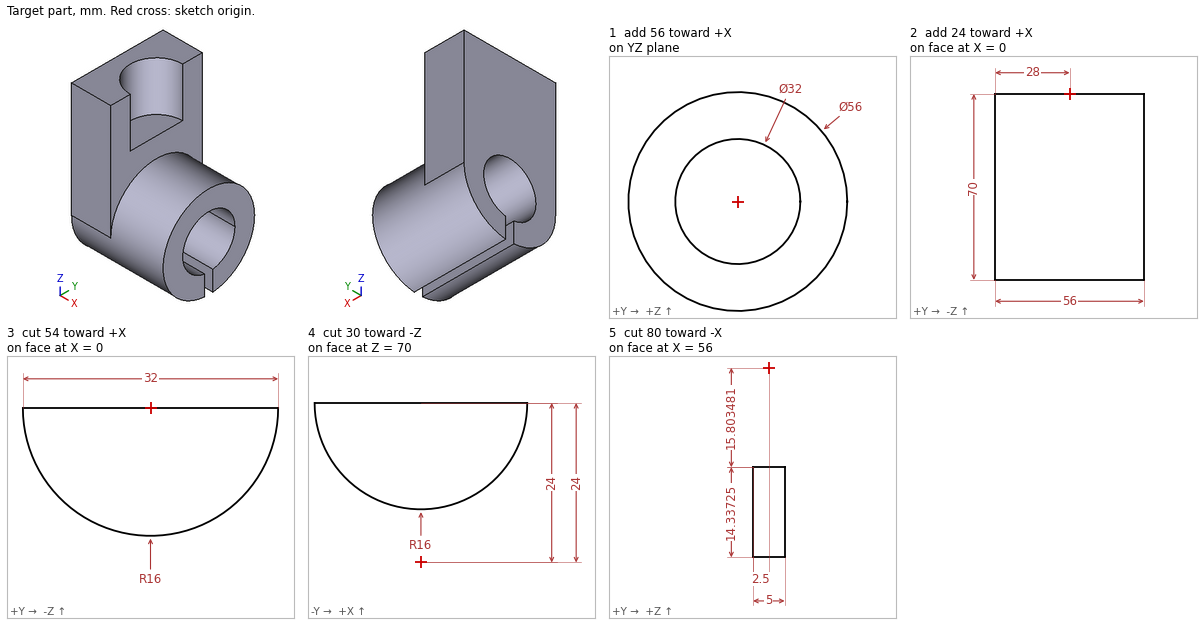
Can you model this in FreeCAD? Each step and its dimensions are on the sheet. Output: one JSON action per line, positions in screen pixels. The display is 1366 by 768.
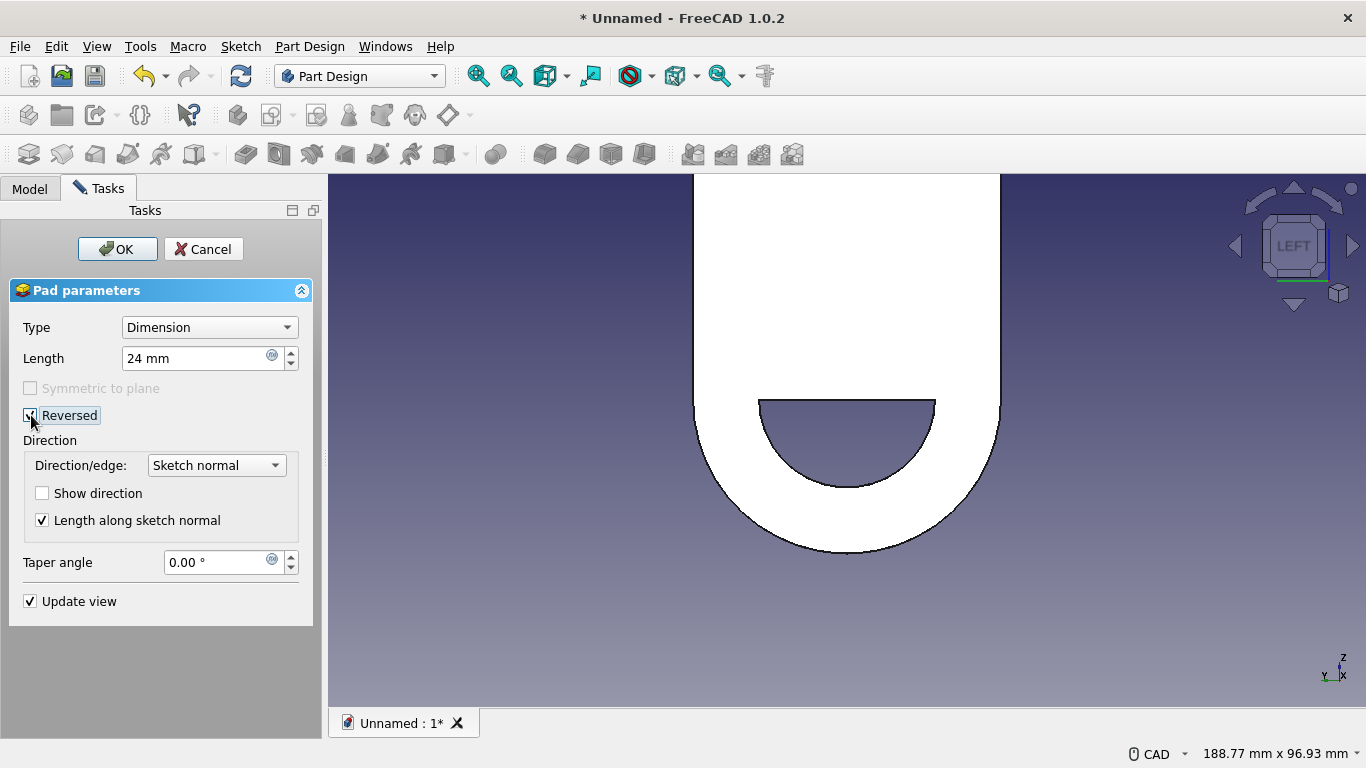
{"action": "left_click", "coordinate": [118, 249]}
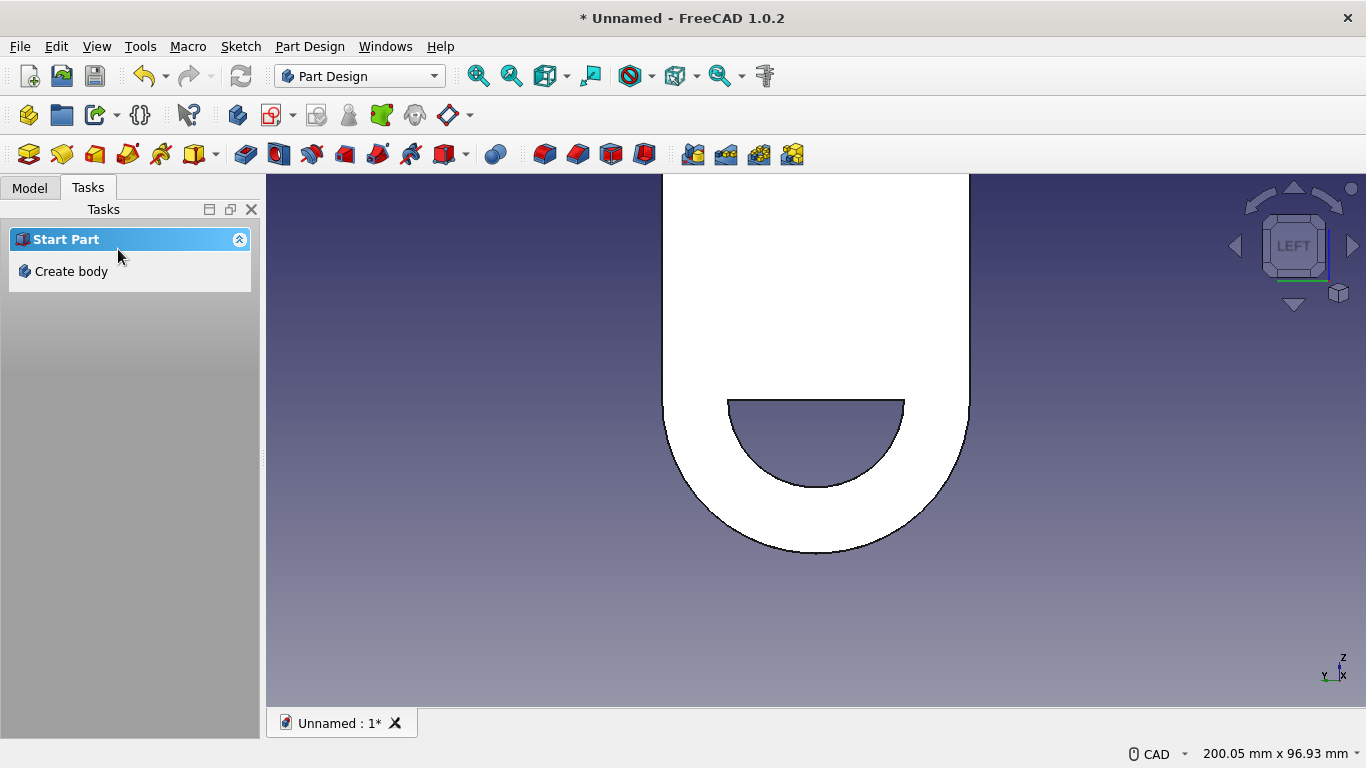
{"action": "left_click", "coordinate": [479, 76]}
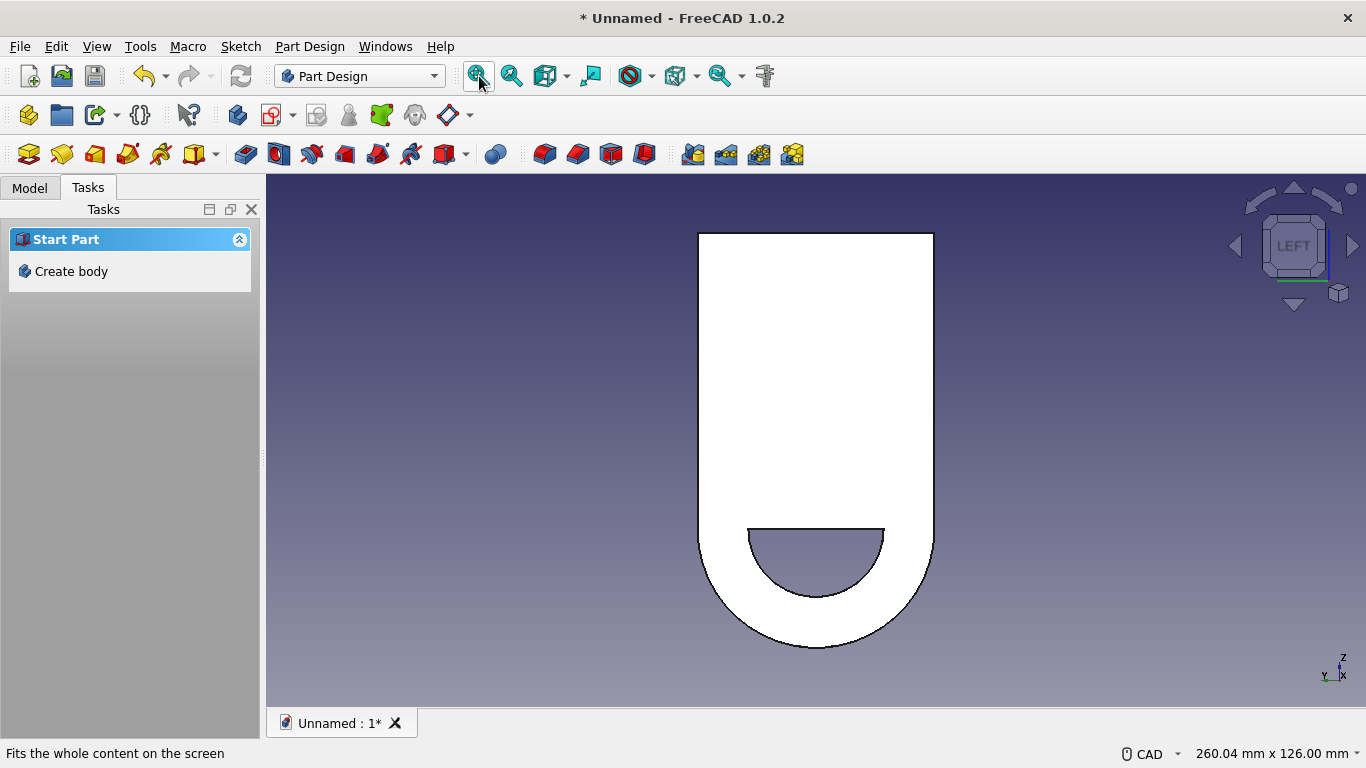
{"action": "left_click", "coordinate": [816, 380]}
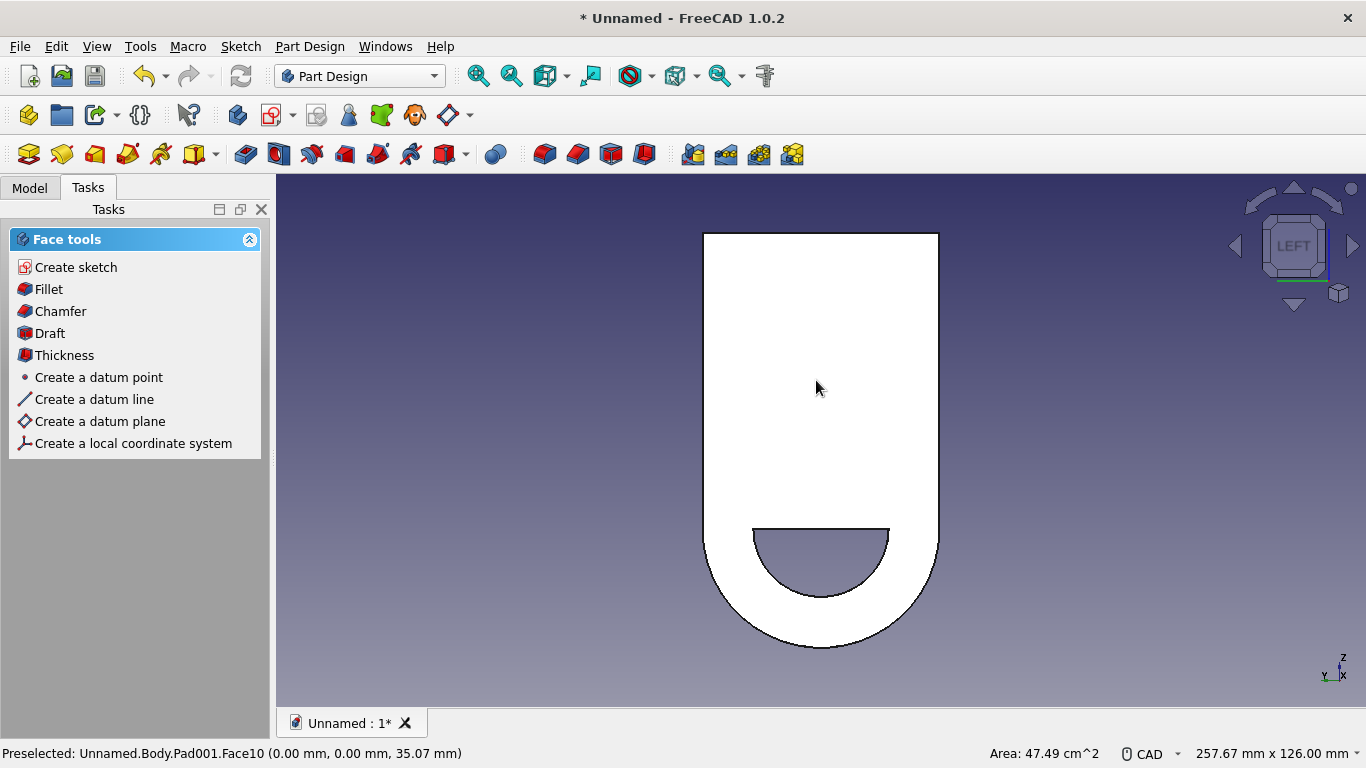
{"action": "left_click", "coordinate": [270, 116]}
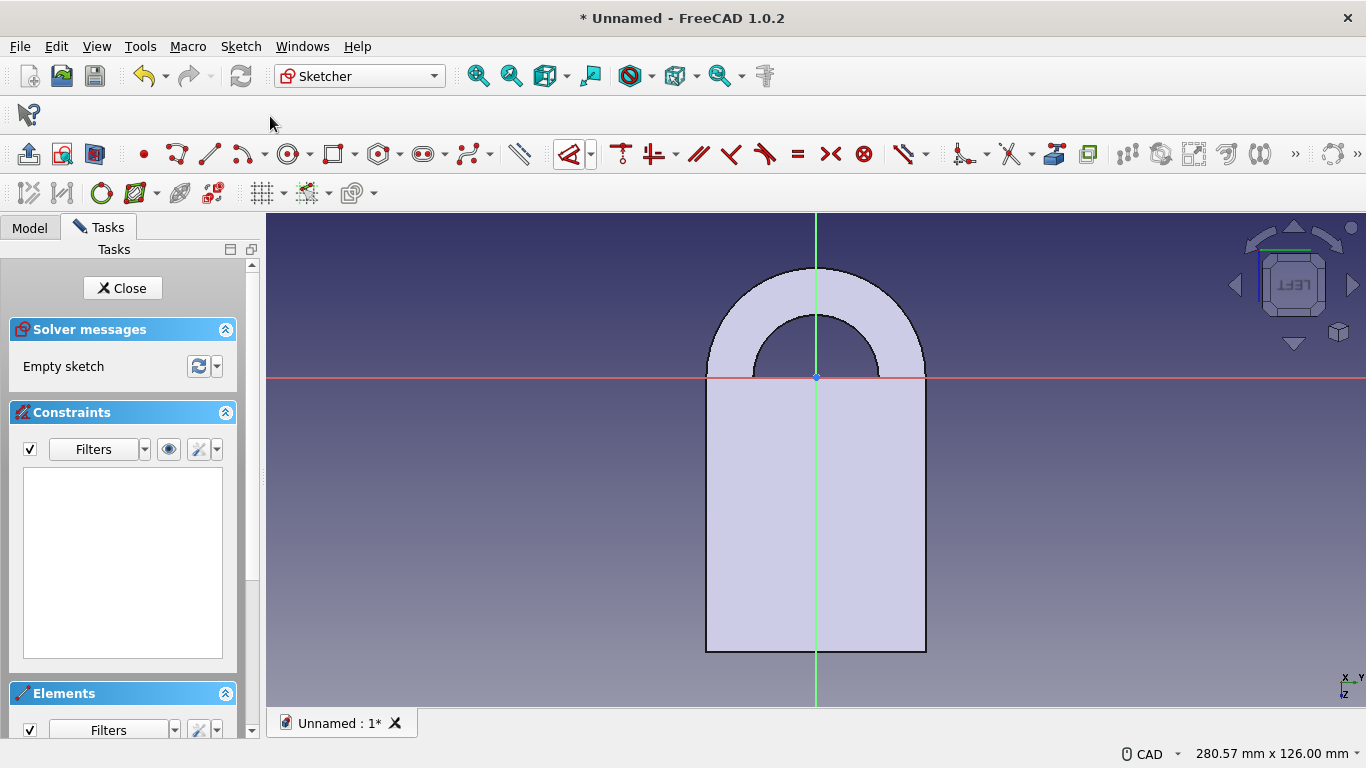
{"action": "scroll", "coordinate": [833, 396], "scroll_direction": "up", "scroll_amount": 8}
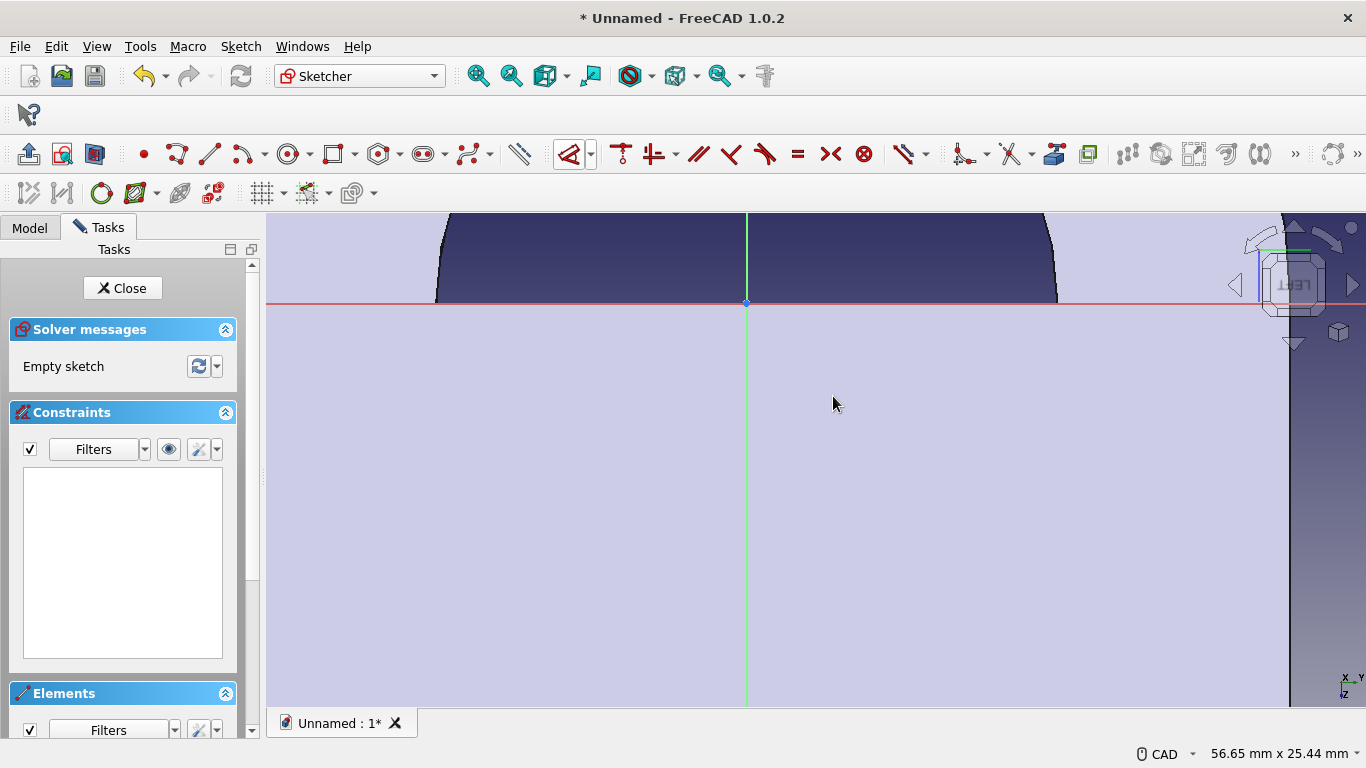
{"action": "left_click", "coordinate": [210, 154]}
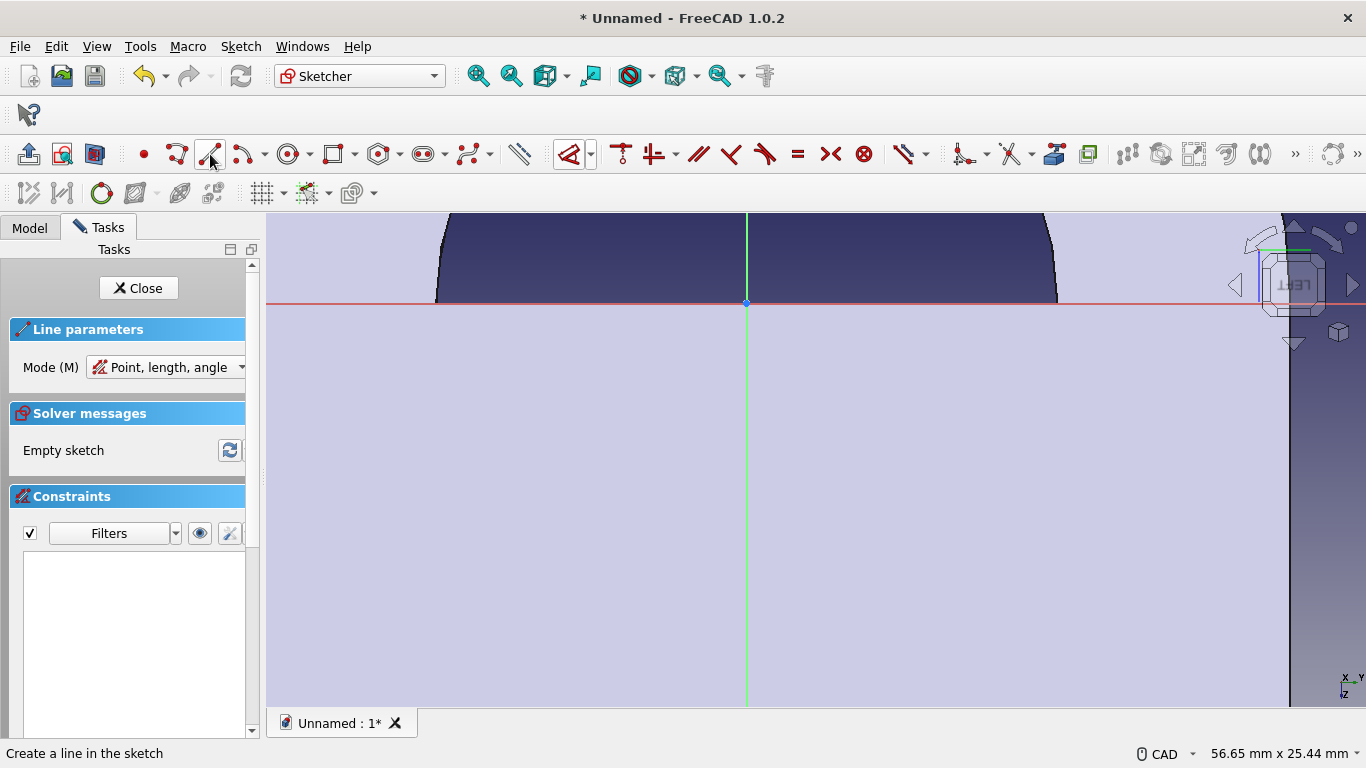
{"action": "left_click", "coordinate": [1057, 304]}
{"action": "left_click", "coordinate": [436, 313]}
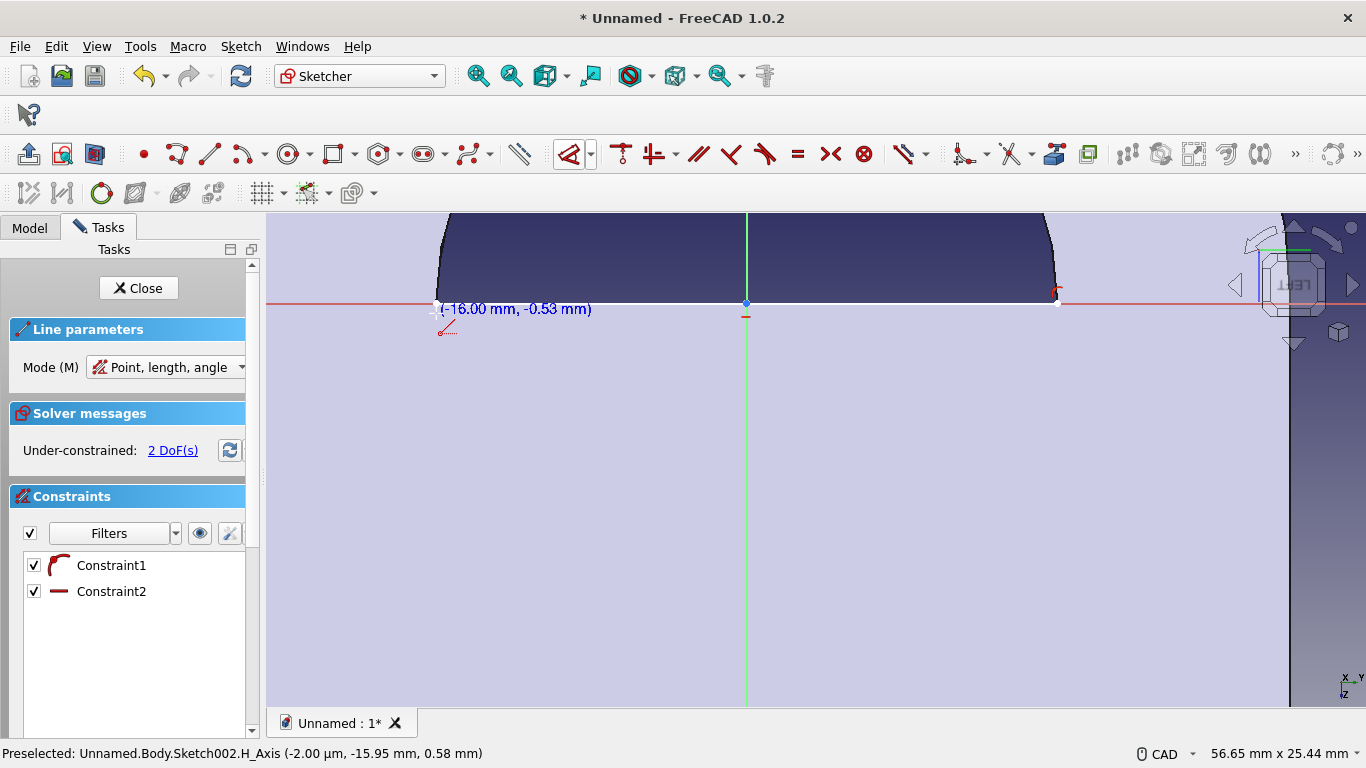
{"action": "left_click", "coordinate": [264, 154]}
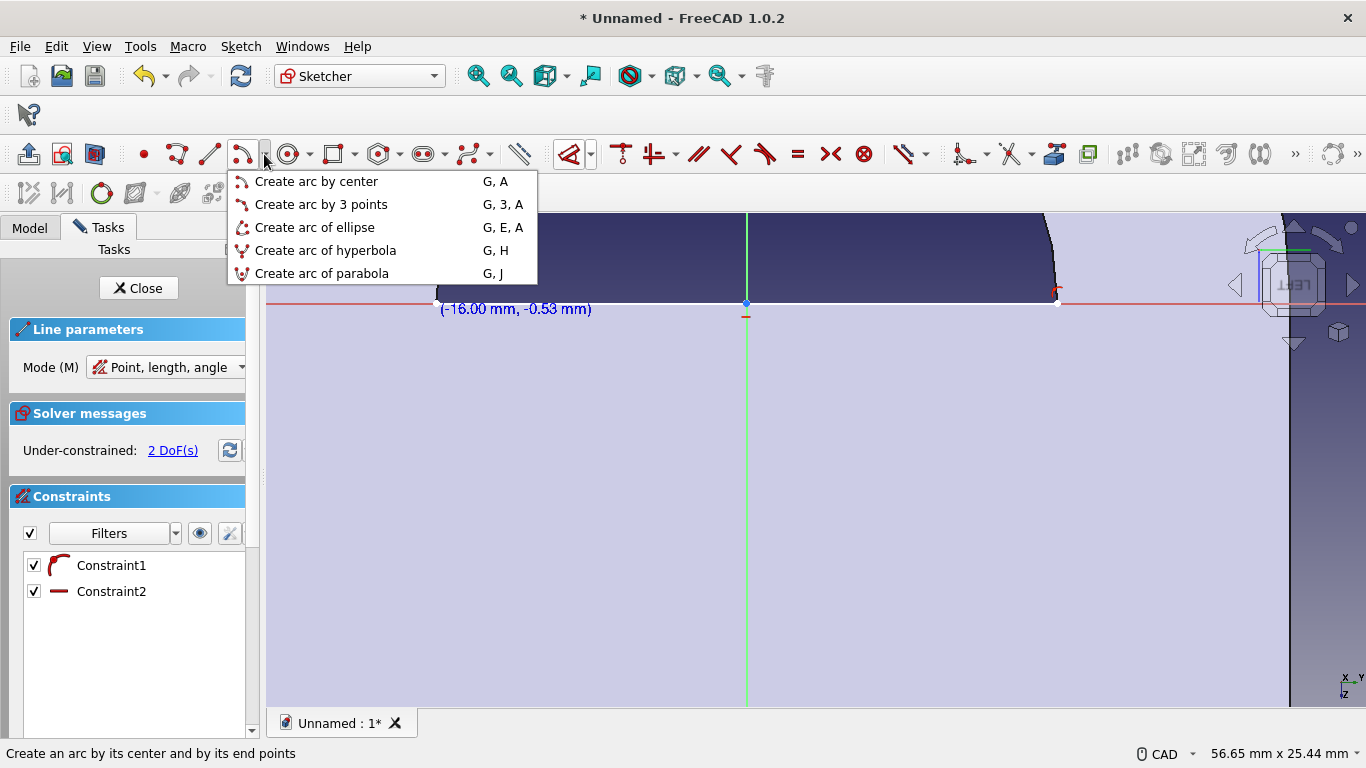
{"action": "left_click", "coordinate": [382, 204]}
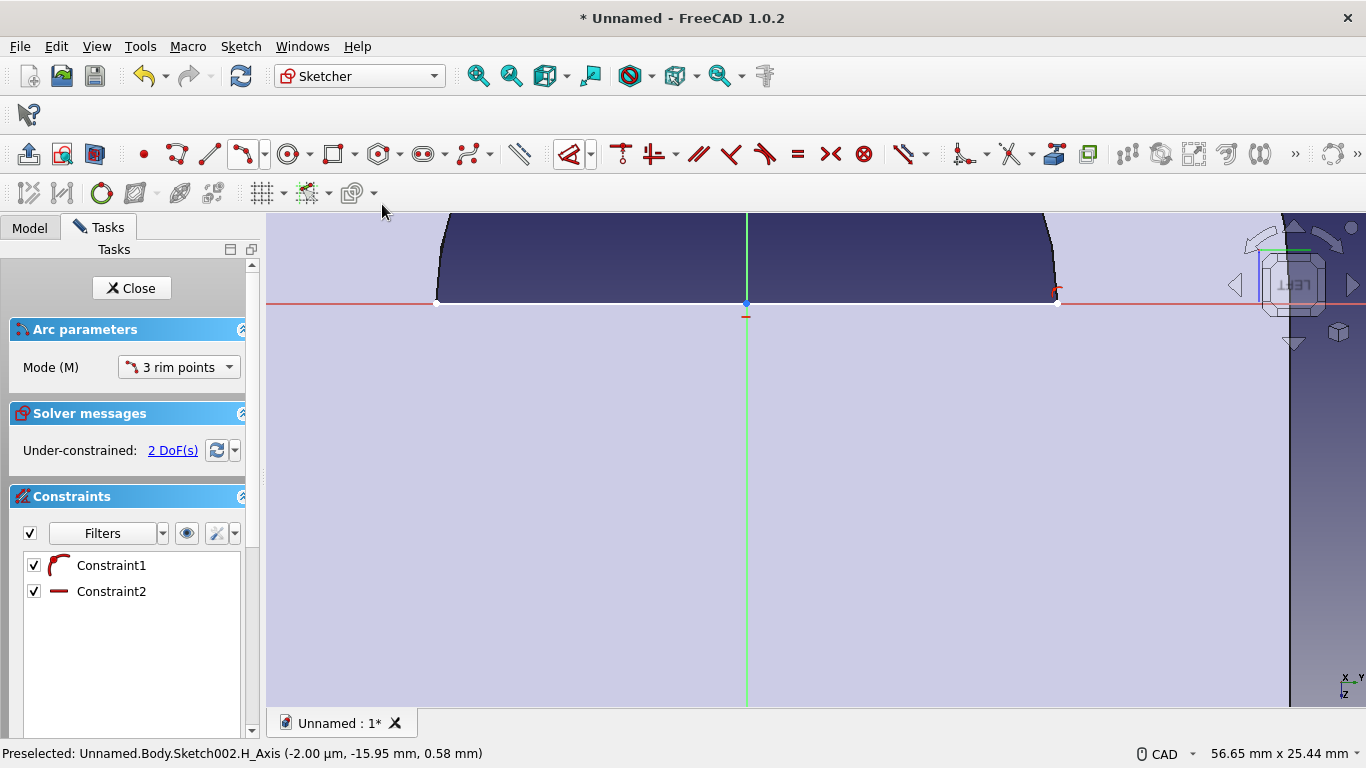
{"action": "left_click", "coordinate": [436, 313]}
{"action": "left_click", "coordinate": [1057, 304]}
{"action": "left_click", "coordinate": [651, 599]}
{"action": "key", "text": "Escape"}